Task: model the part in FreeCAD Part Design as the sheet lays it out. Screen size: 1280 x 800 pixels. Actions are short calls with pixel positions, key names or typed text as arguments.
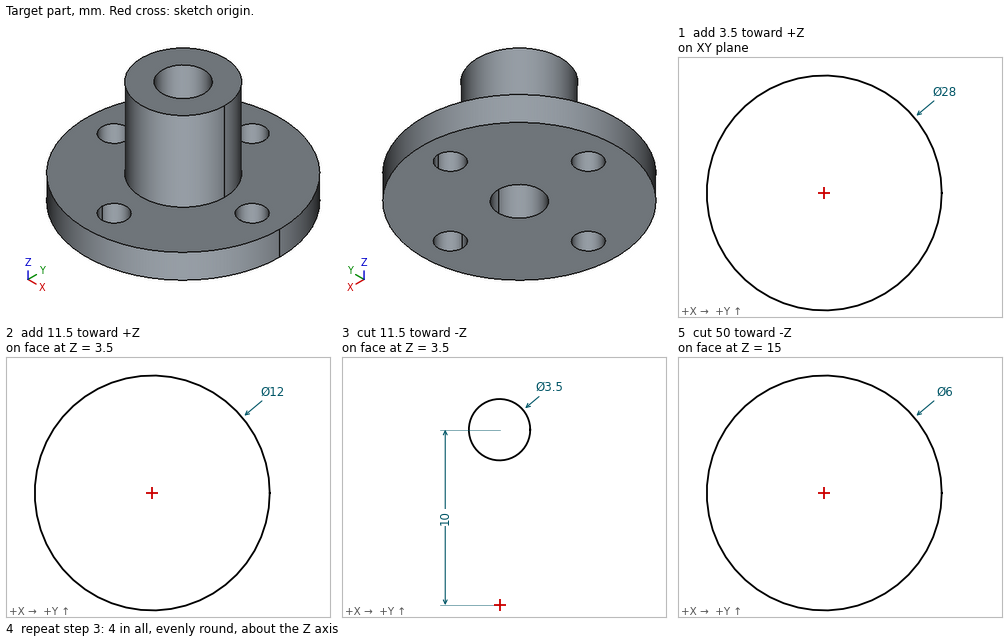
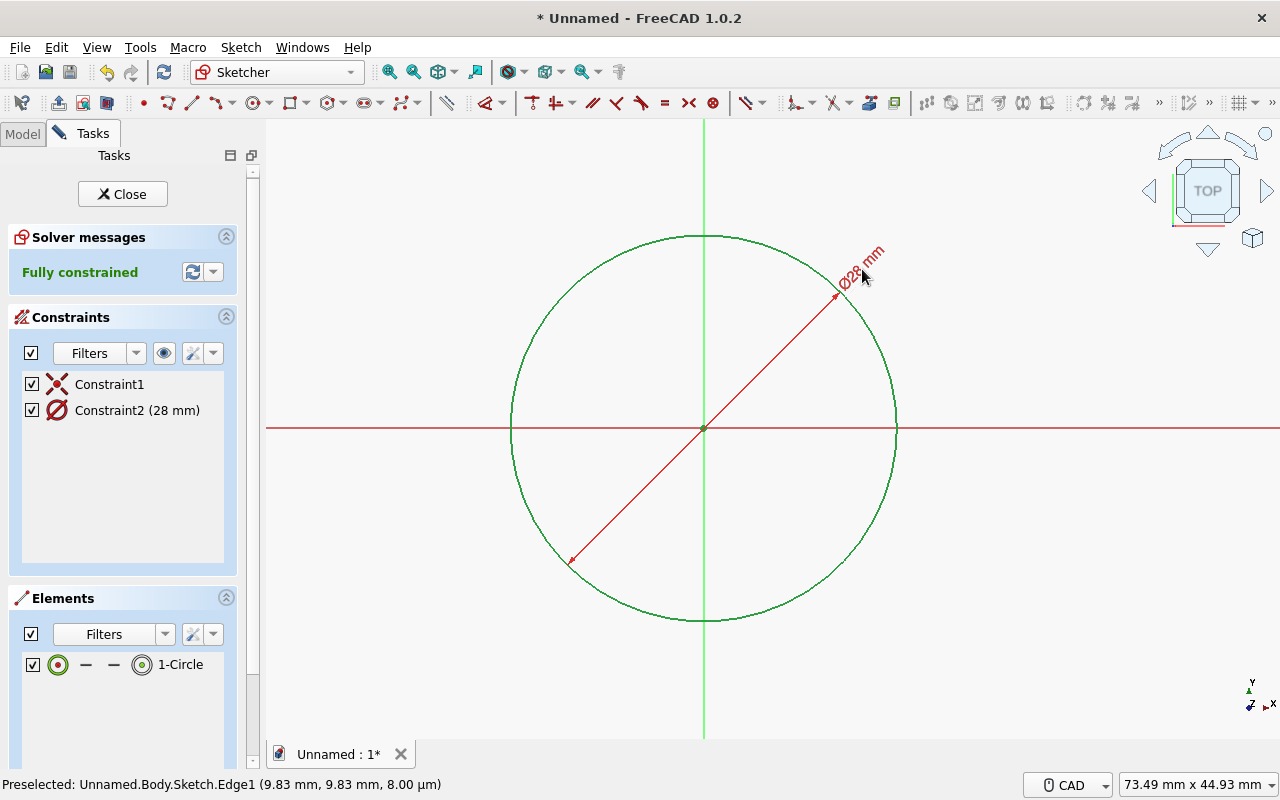
click(123, 194)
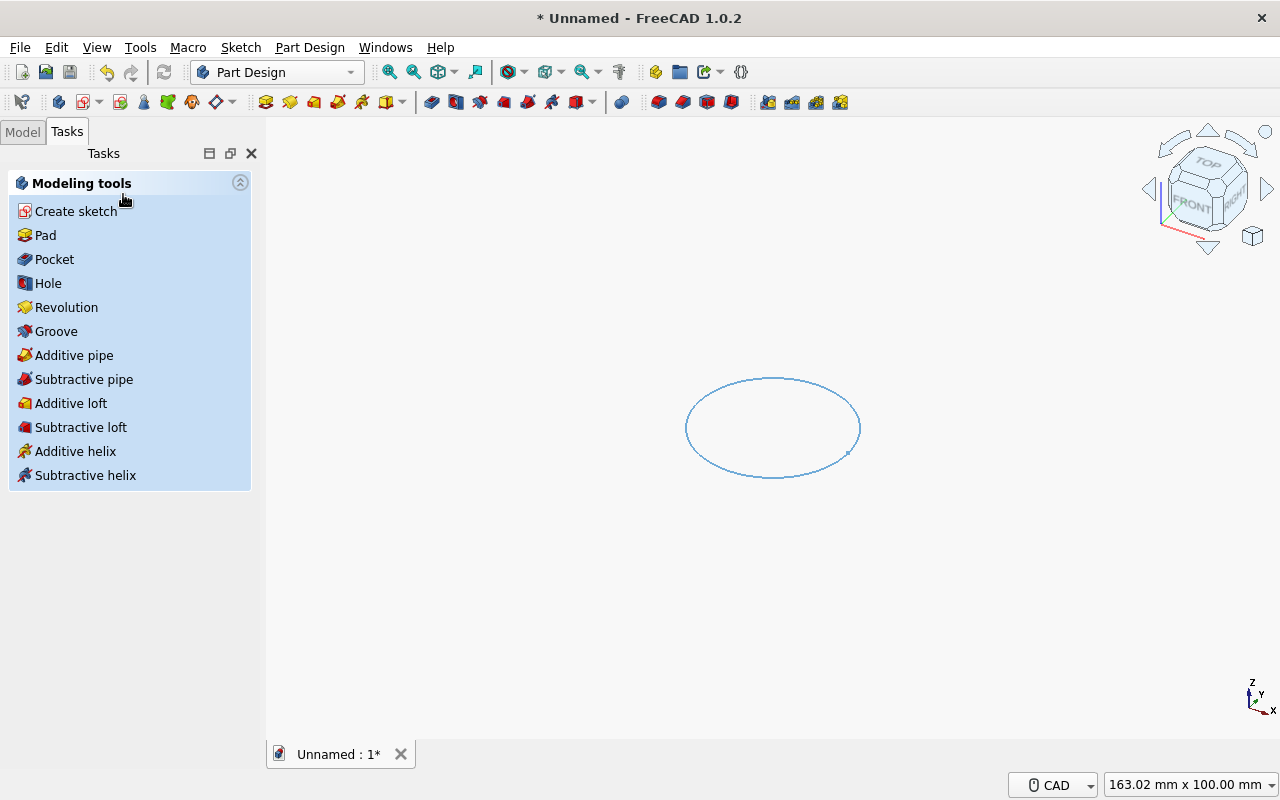
click(266, 102)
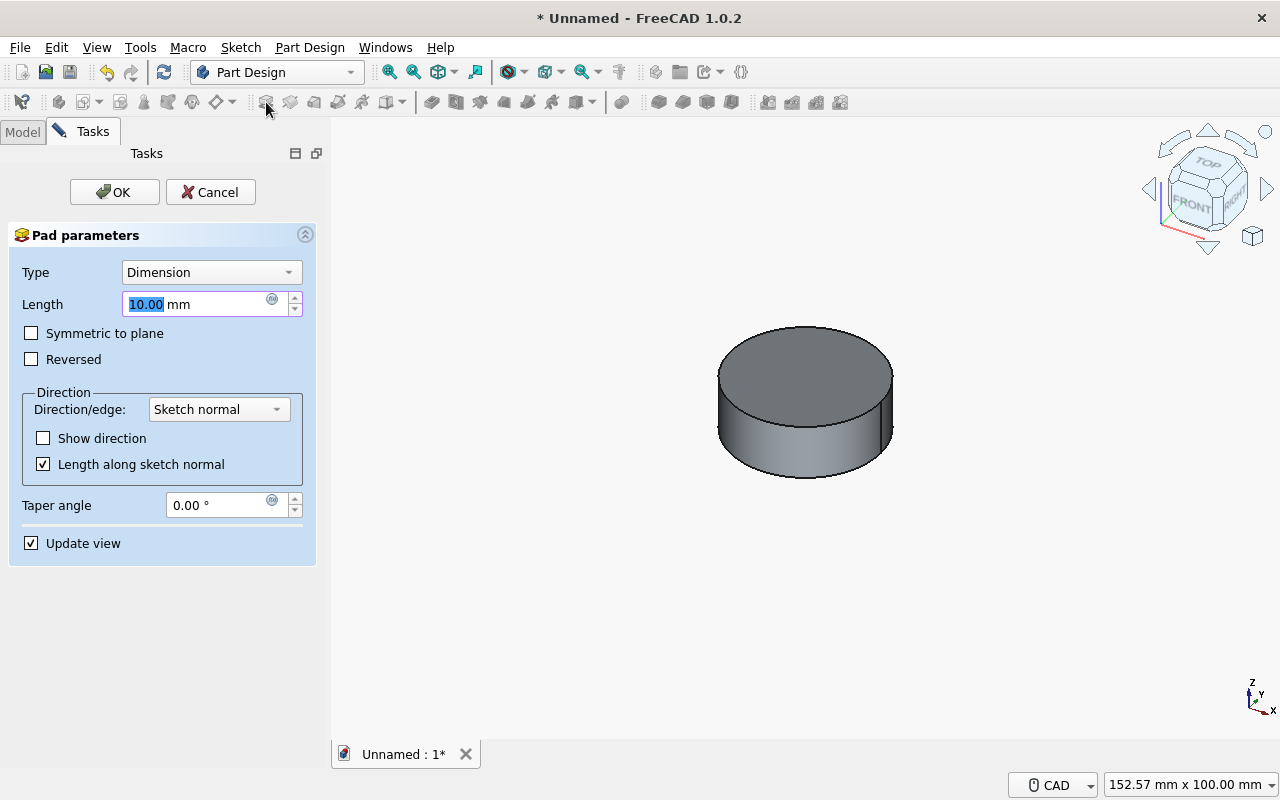
text(3.5)
key(Tab)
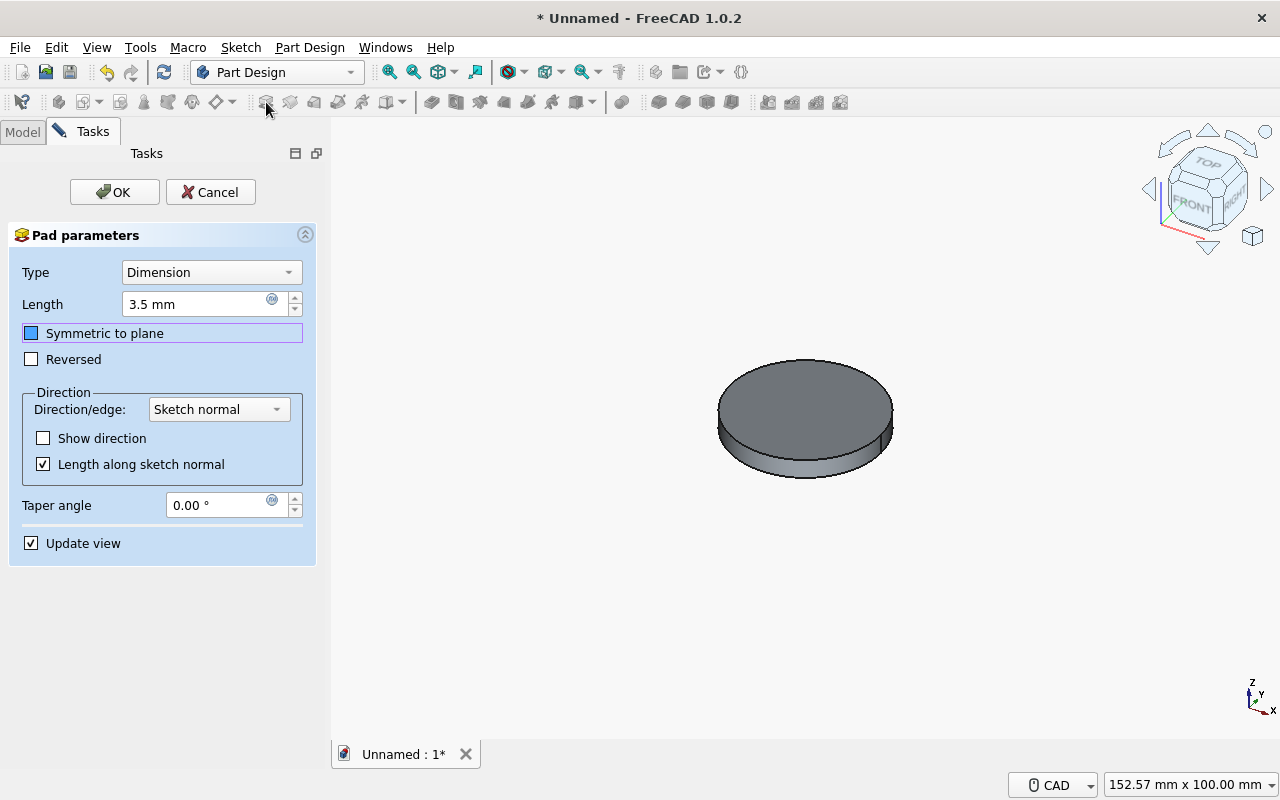
click(115, 192)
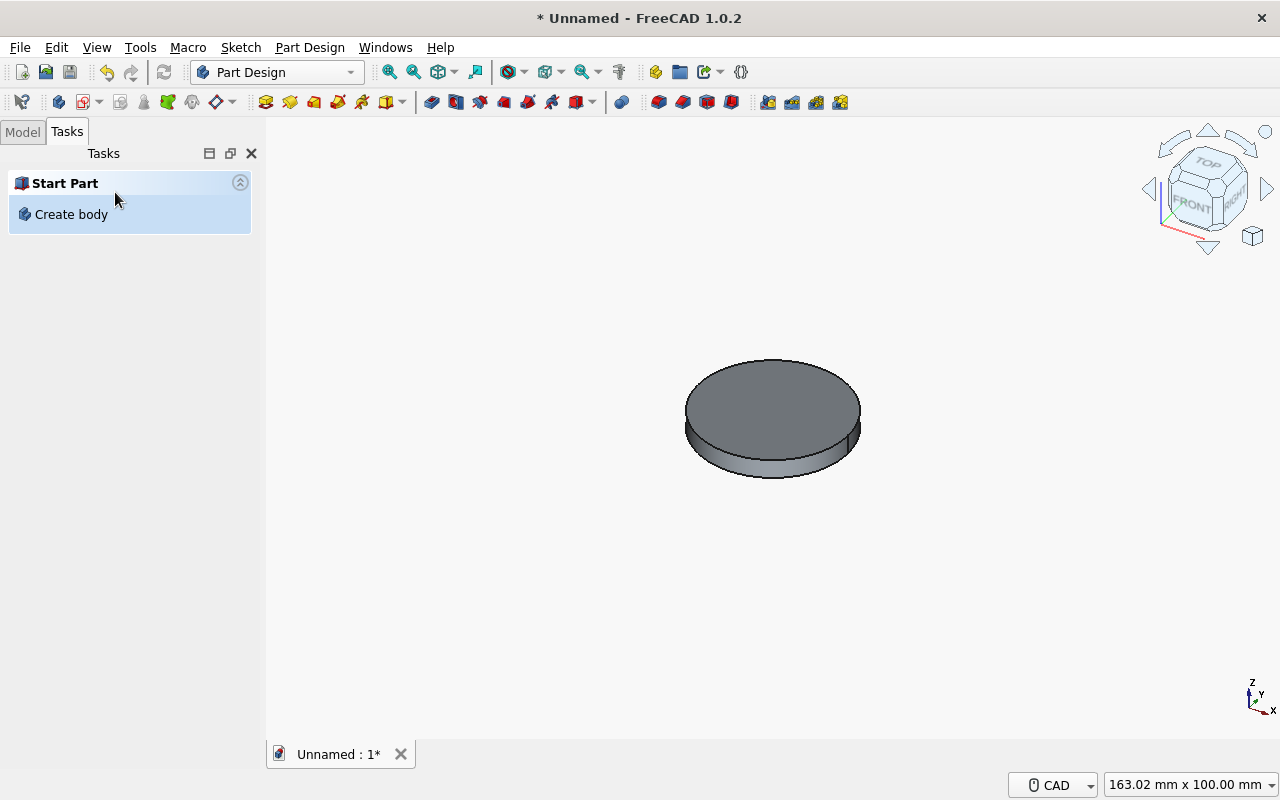
key(v)
key(f)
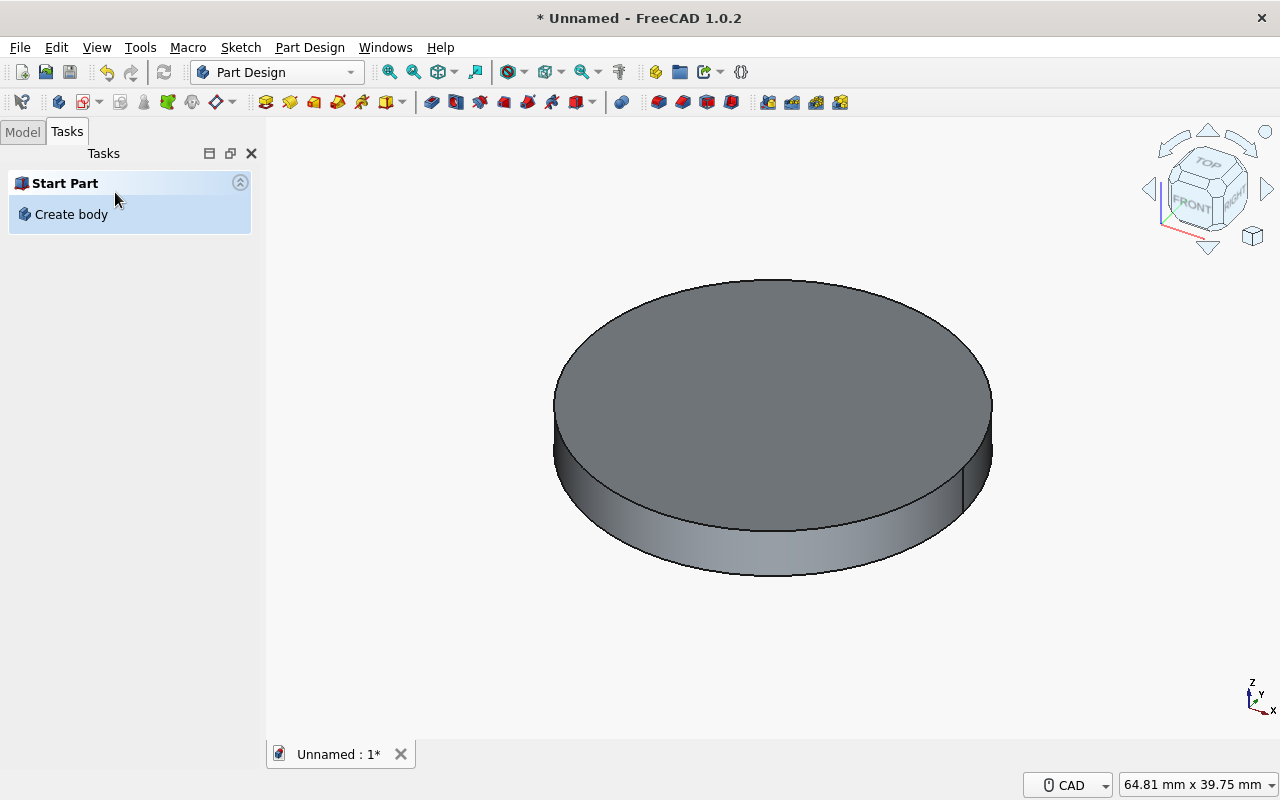
click(773, 405)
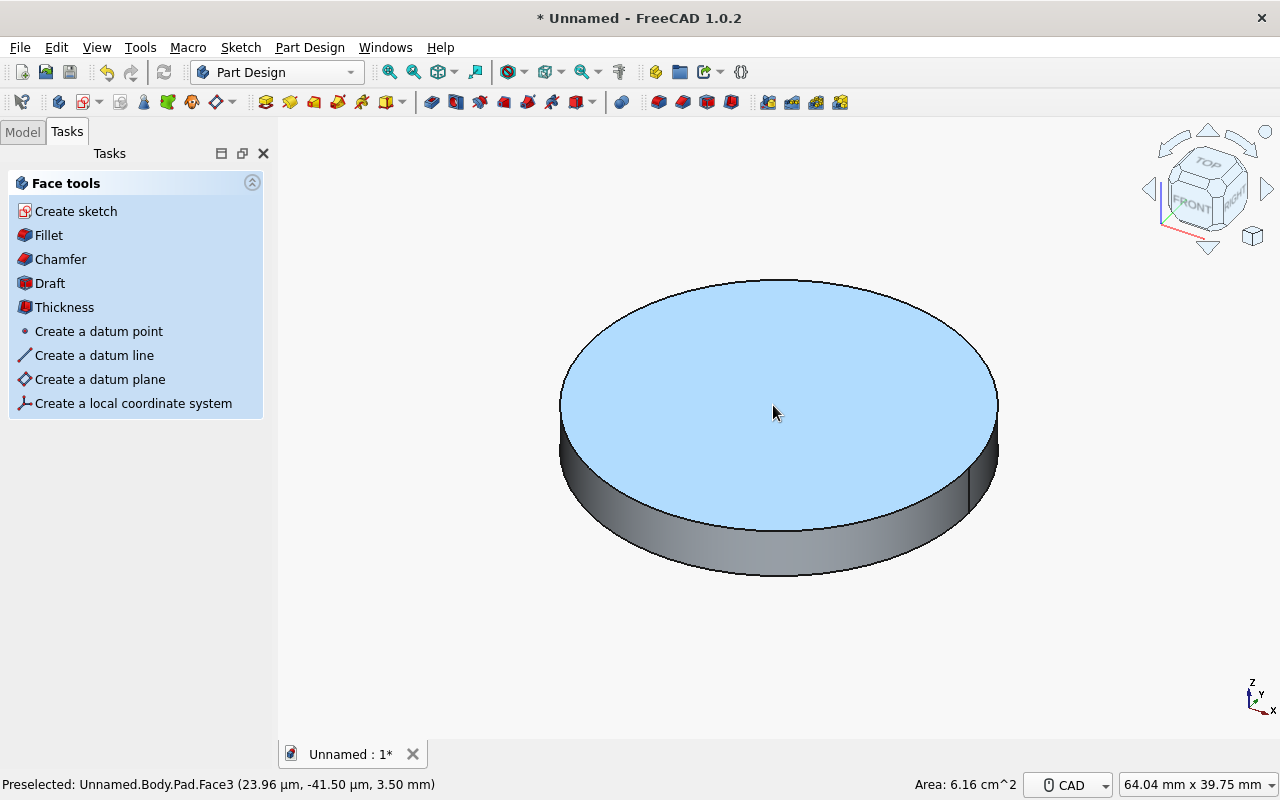
click(84, 102)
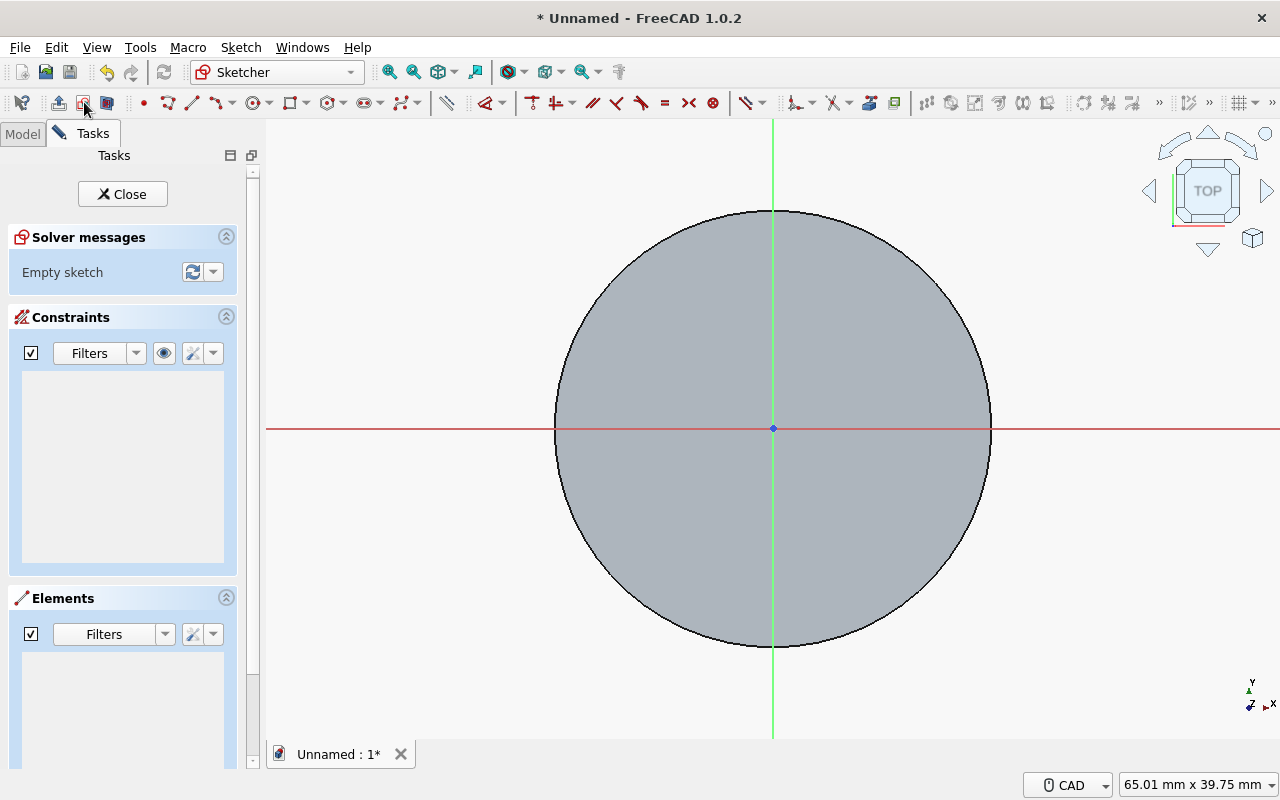
scroll(829, 429, up, 4)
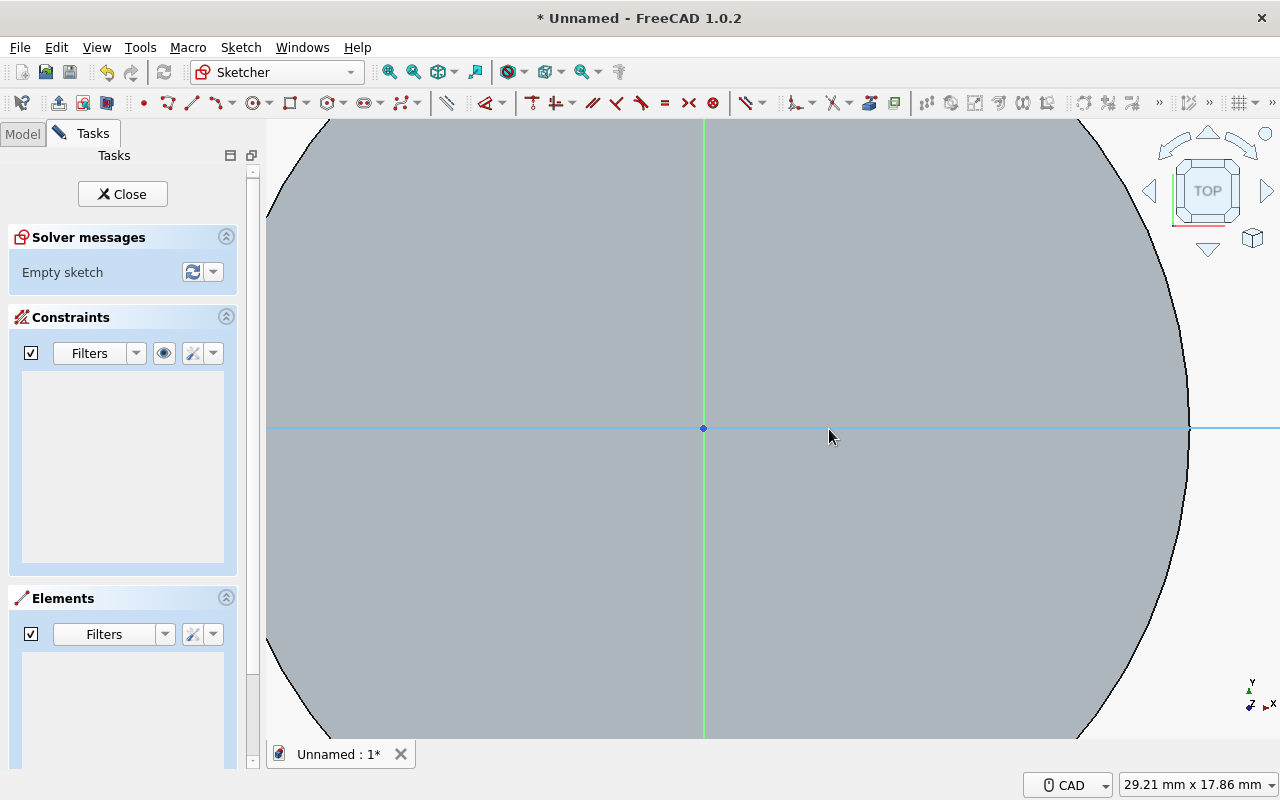
key(g)
key(c)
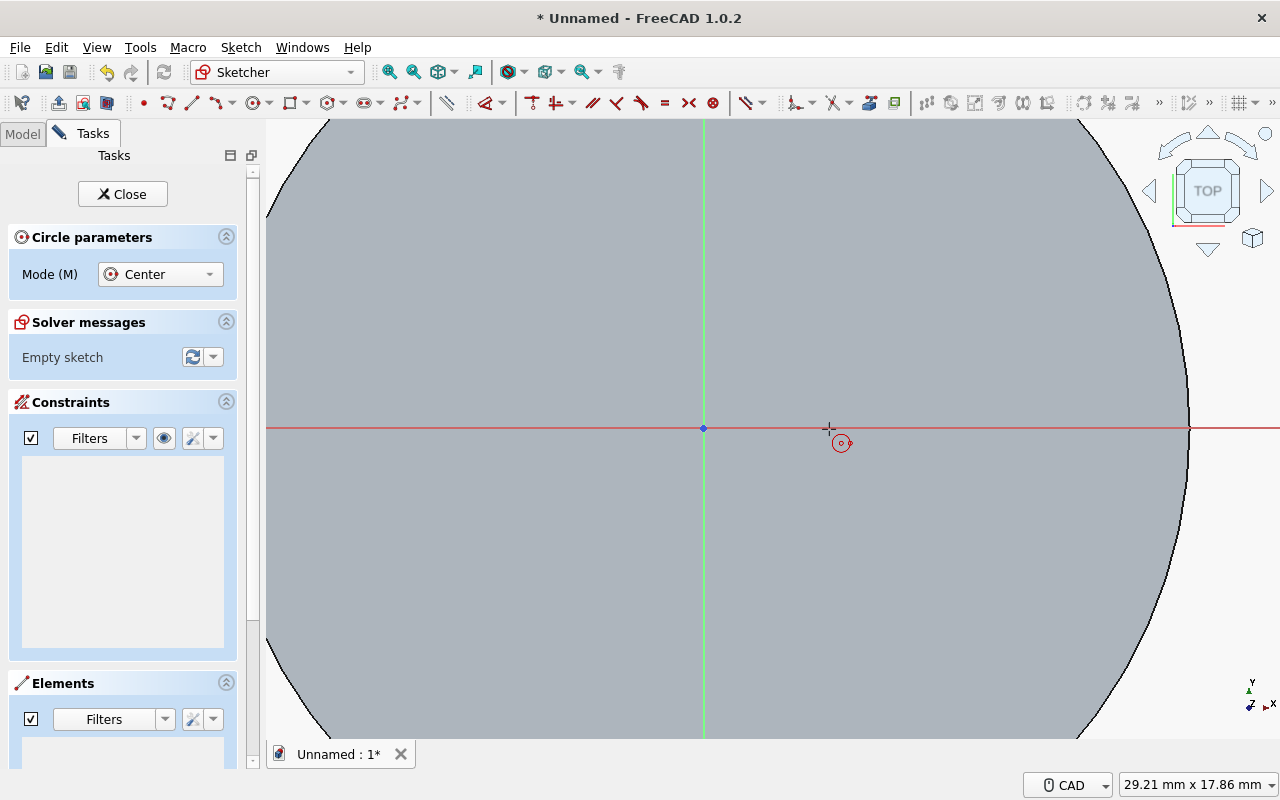
click(704, 428)
click(851, 281)
key(Escape)